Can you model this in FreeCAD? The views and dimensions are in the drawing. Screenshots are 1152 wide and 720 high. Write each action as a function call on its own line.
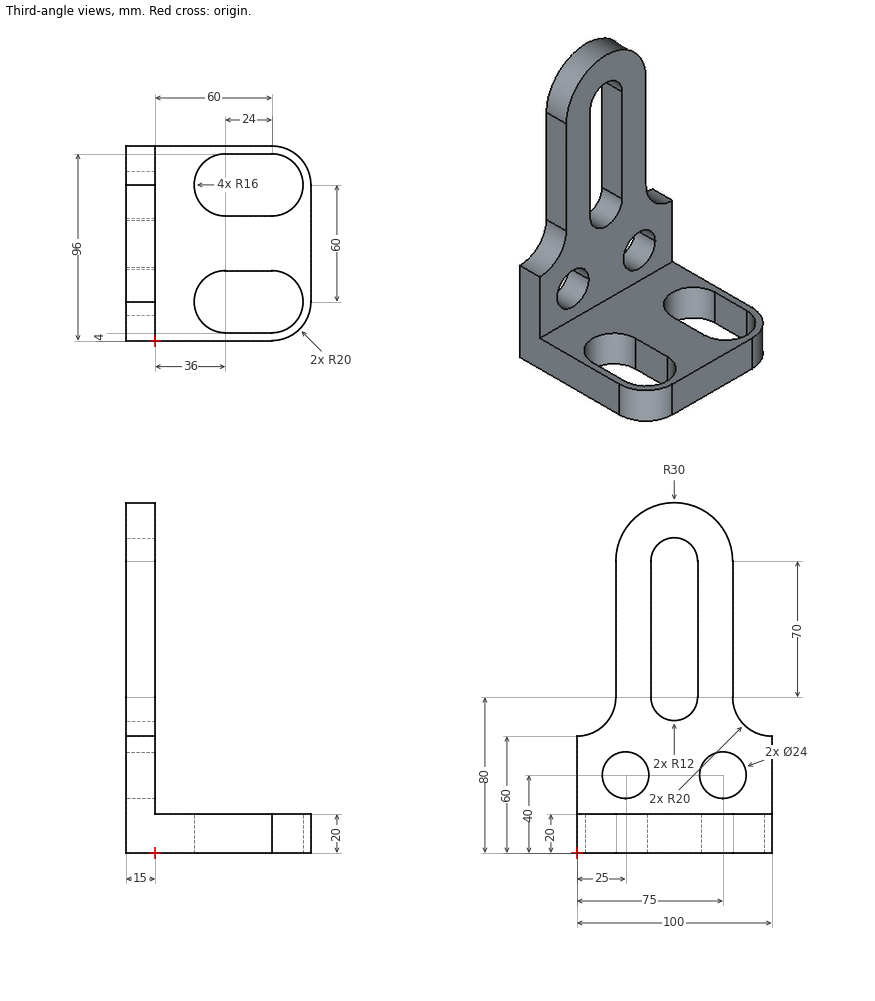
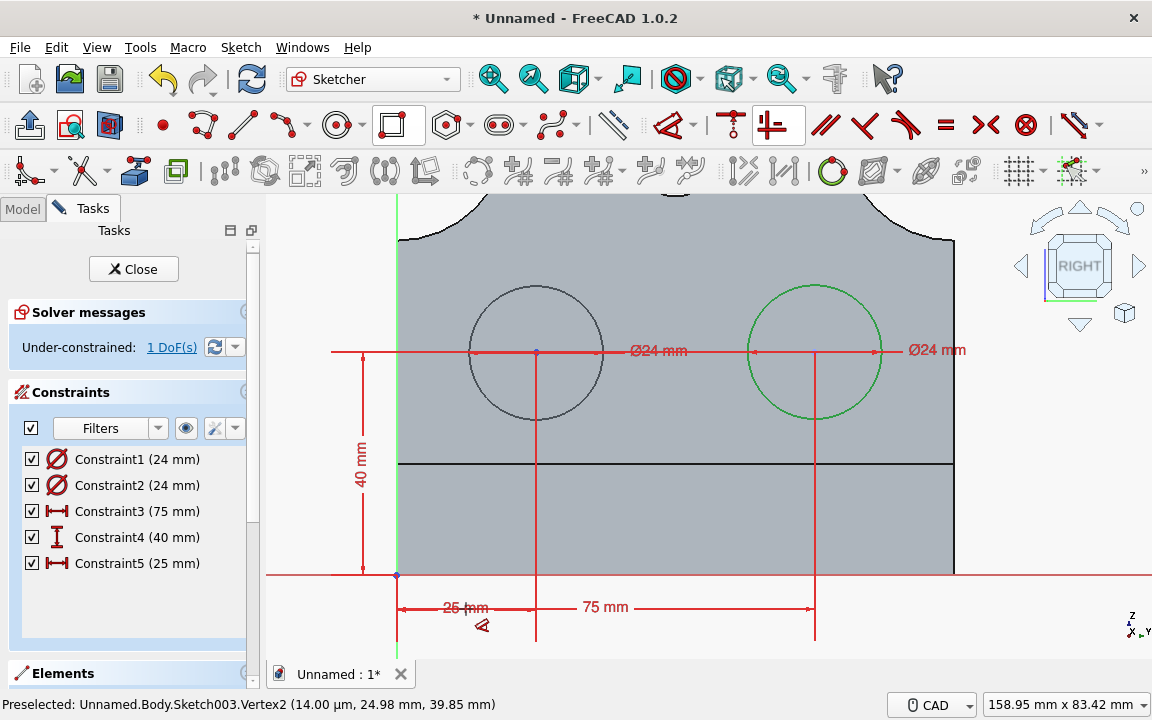
click(536, 353)
click(363, 413)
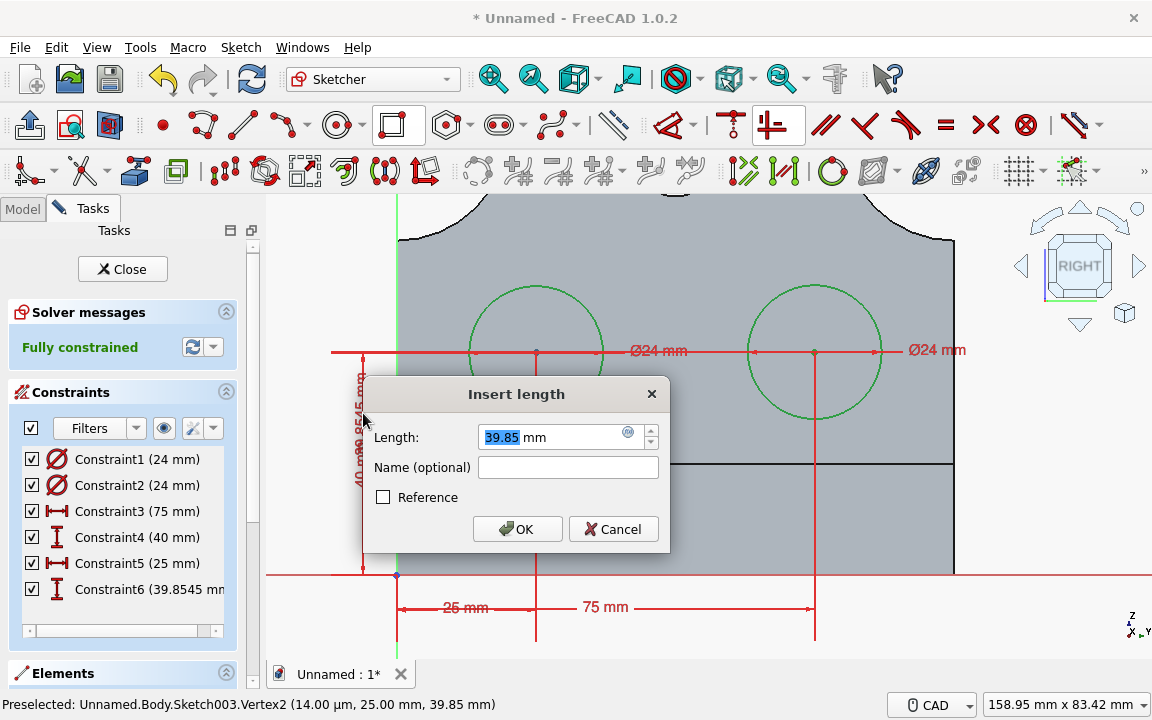
text(40)
key(Return)
key(Escape)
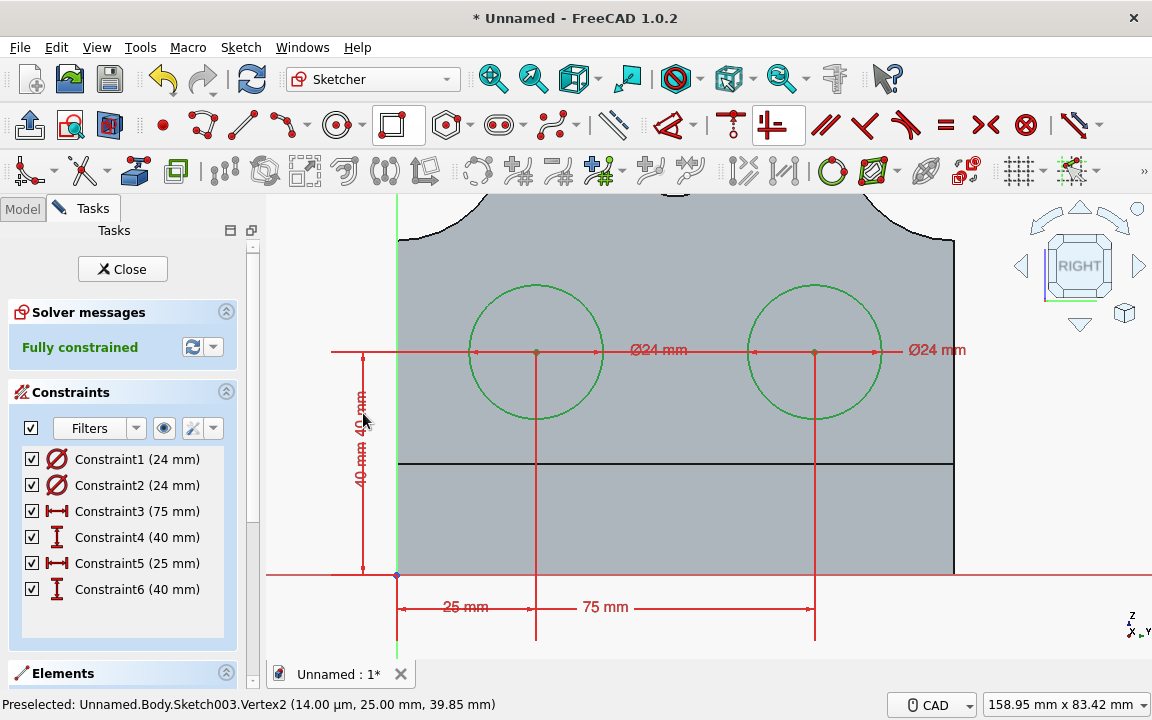
click(123, 269)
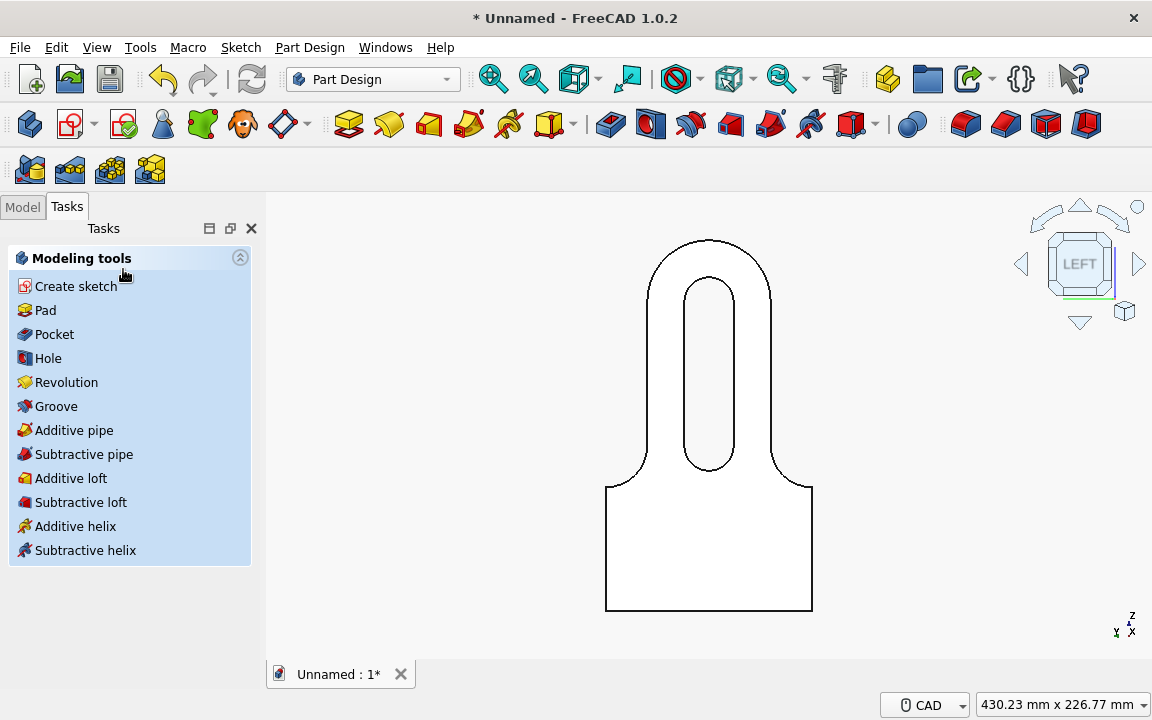
click(612, 124)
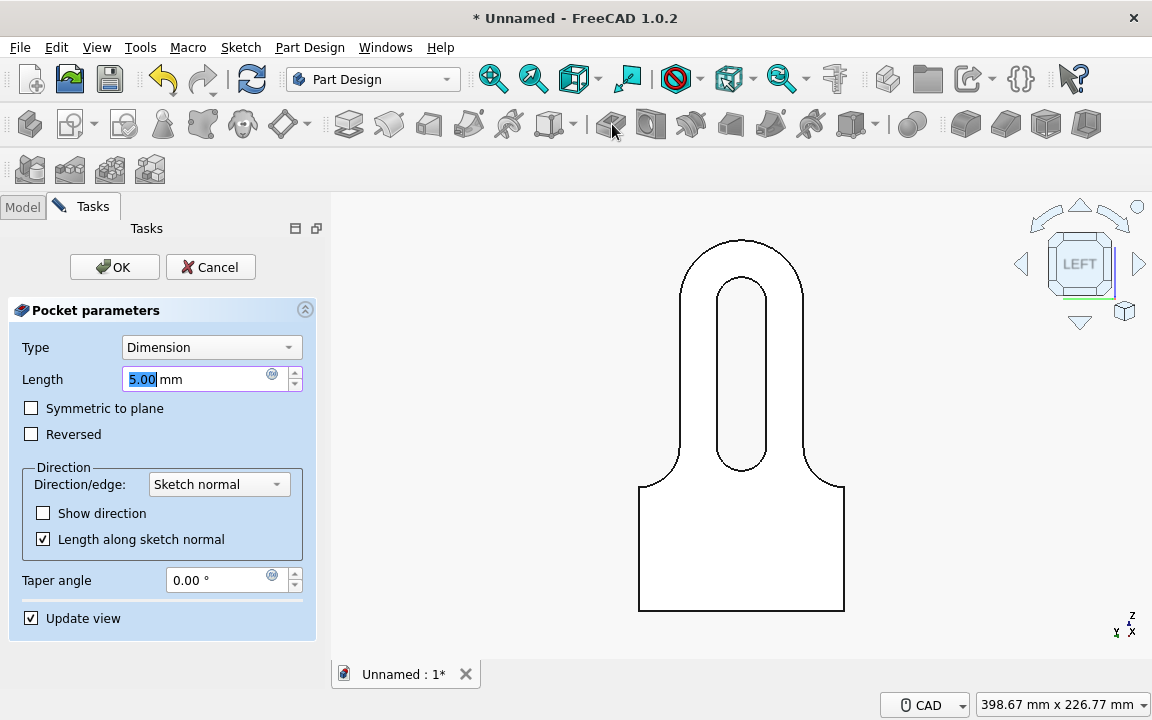
text(15)
key(Tab)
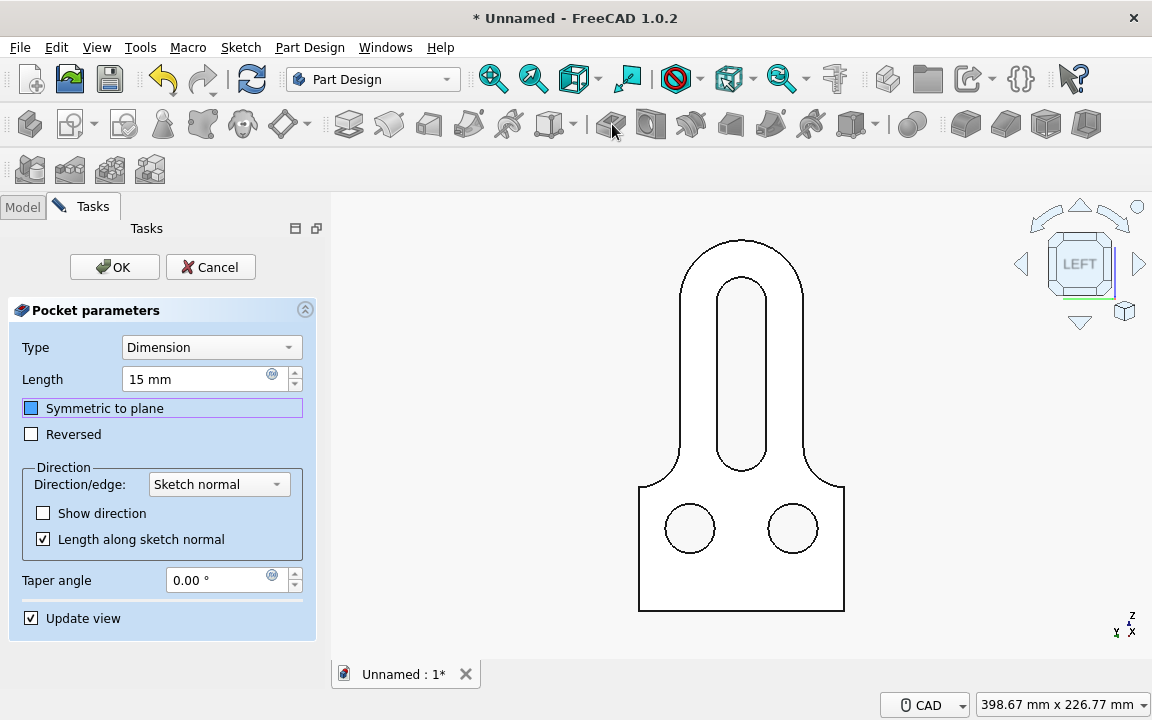
click(115, 267)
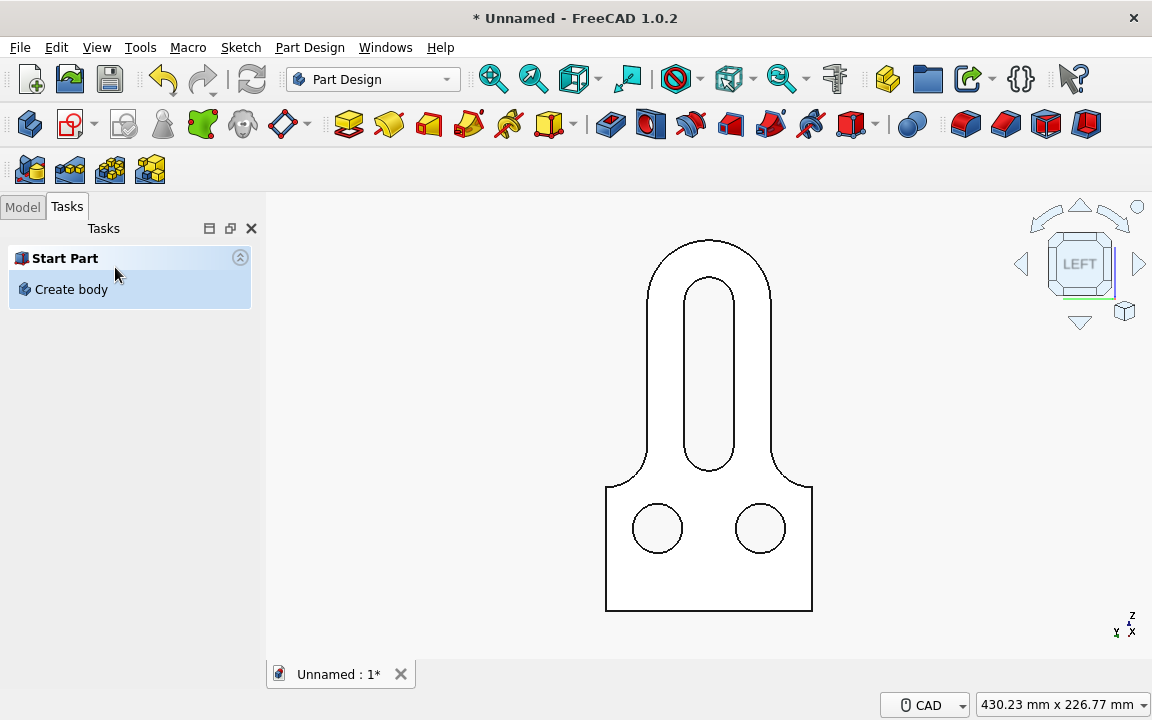
key(0)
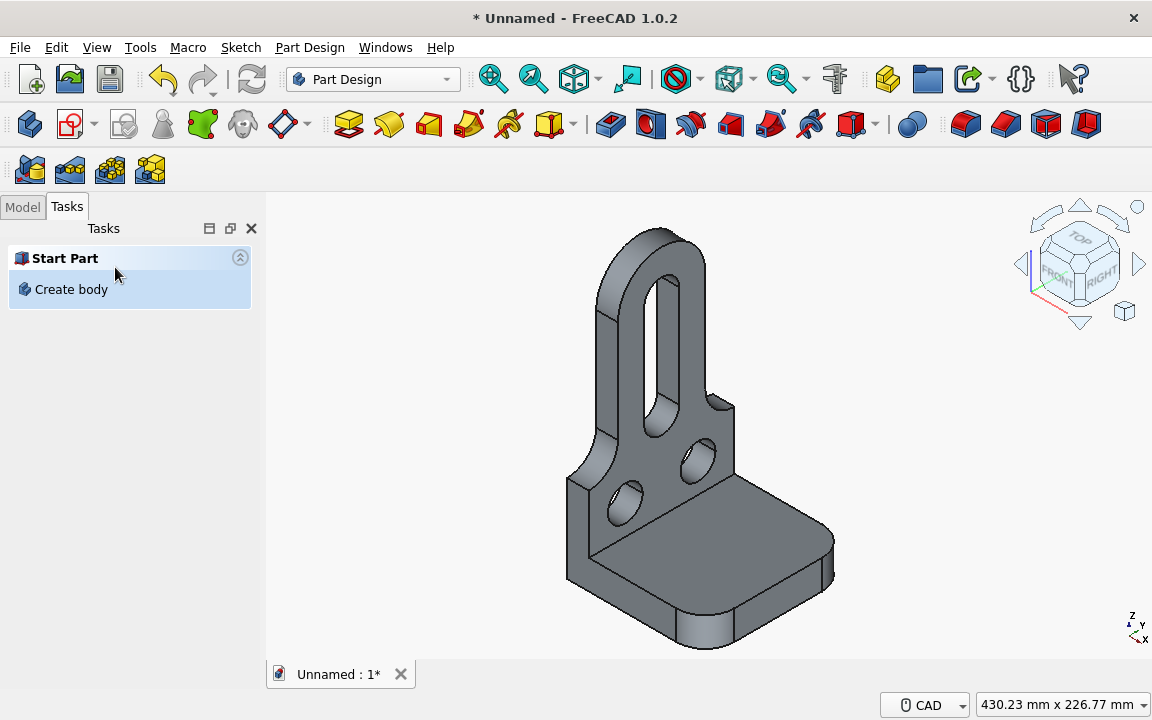
key(v)
key(f)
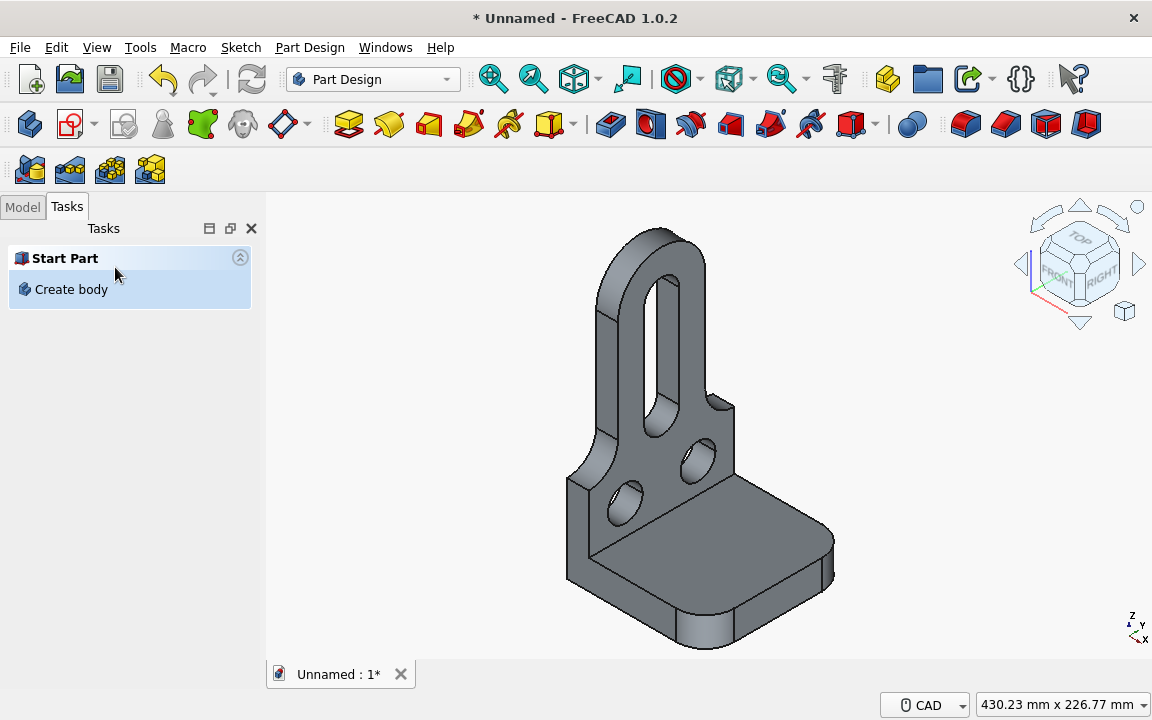
click(720, 549)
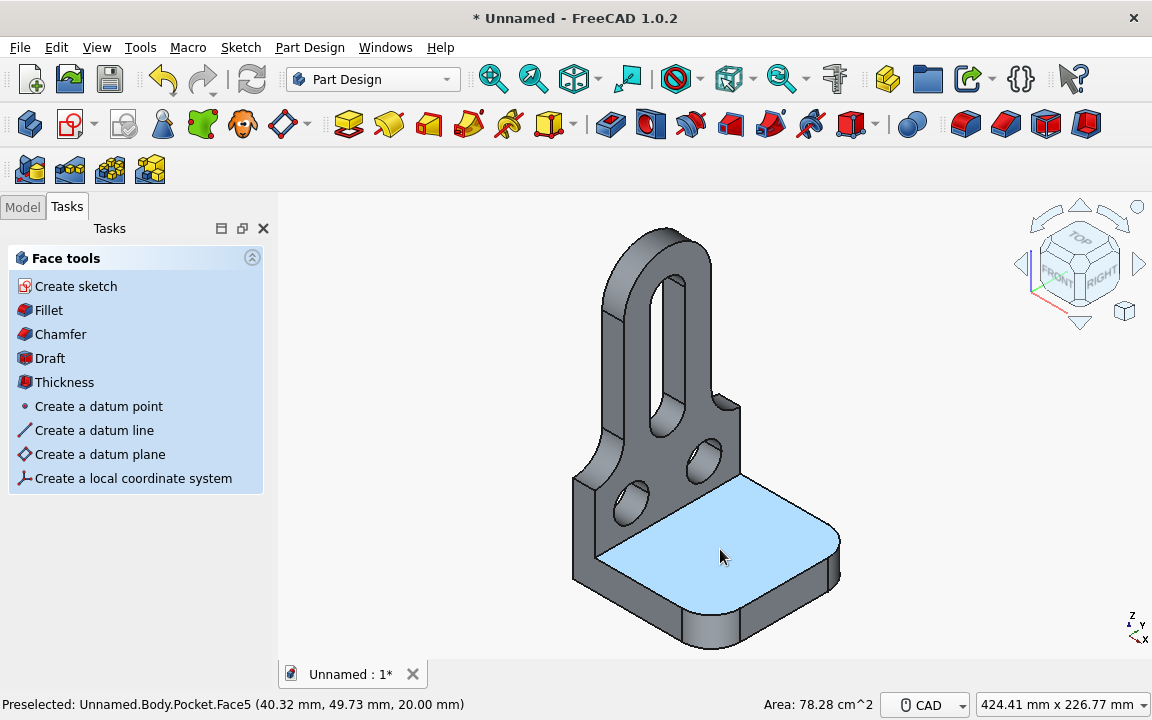
click(70, 124)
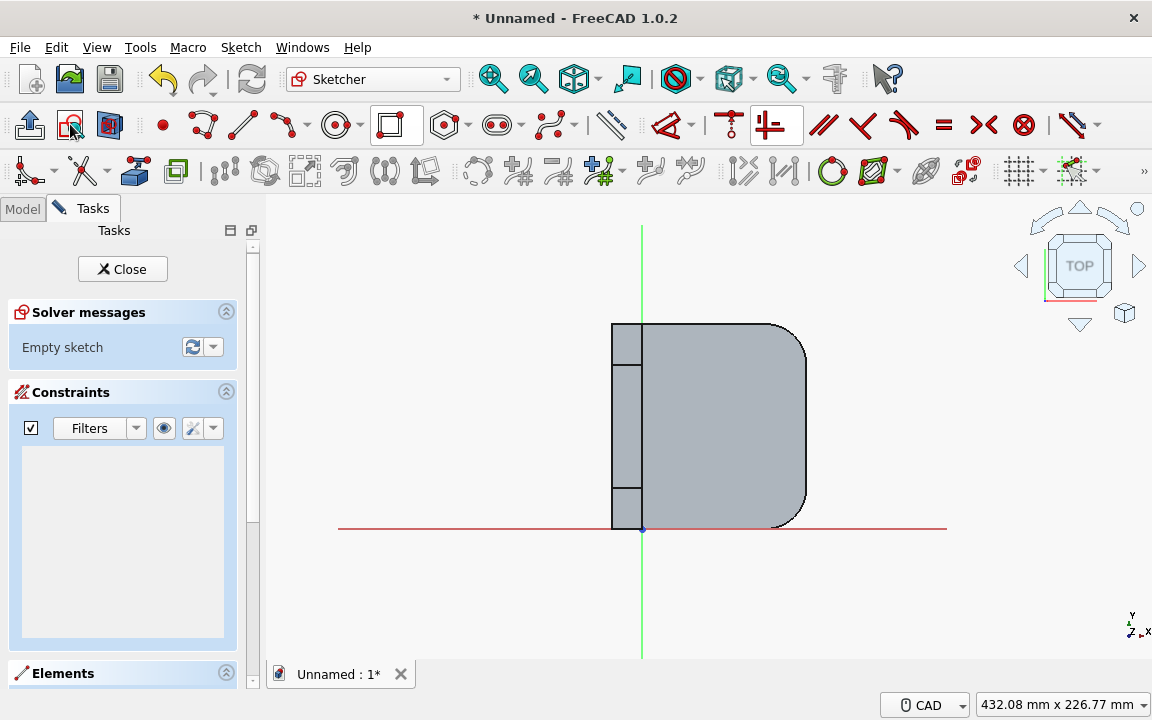
scroll(882, 439, up, 2)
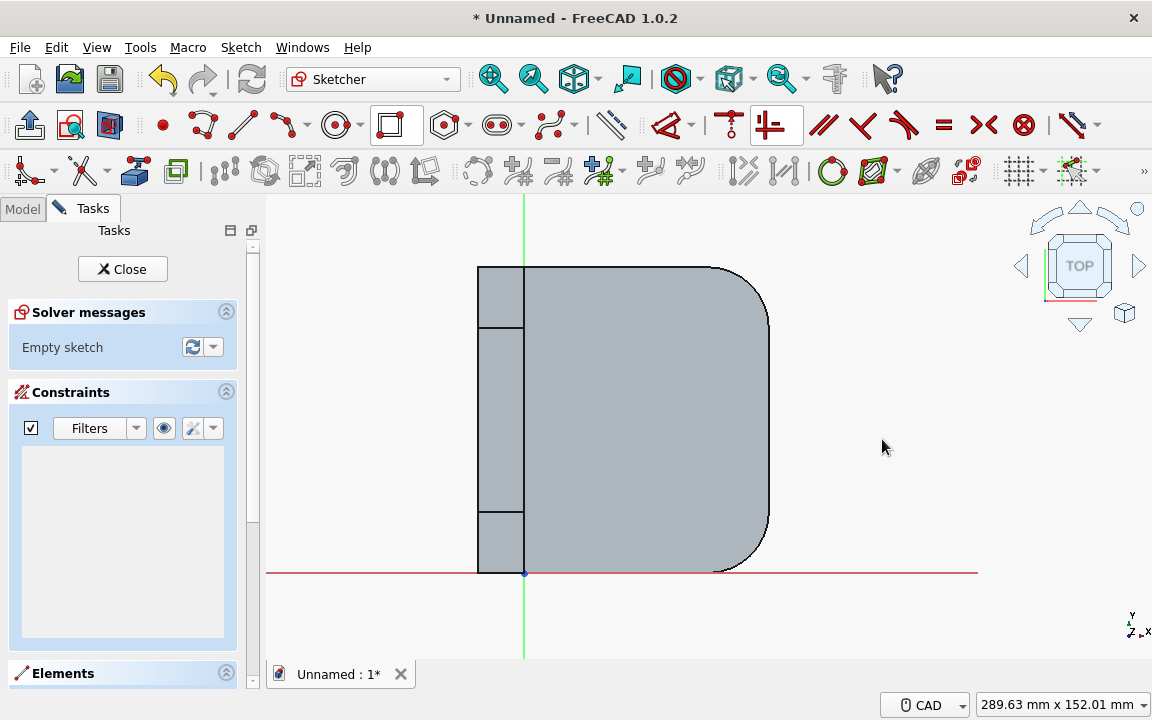
key(g)
key(s)